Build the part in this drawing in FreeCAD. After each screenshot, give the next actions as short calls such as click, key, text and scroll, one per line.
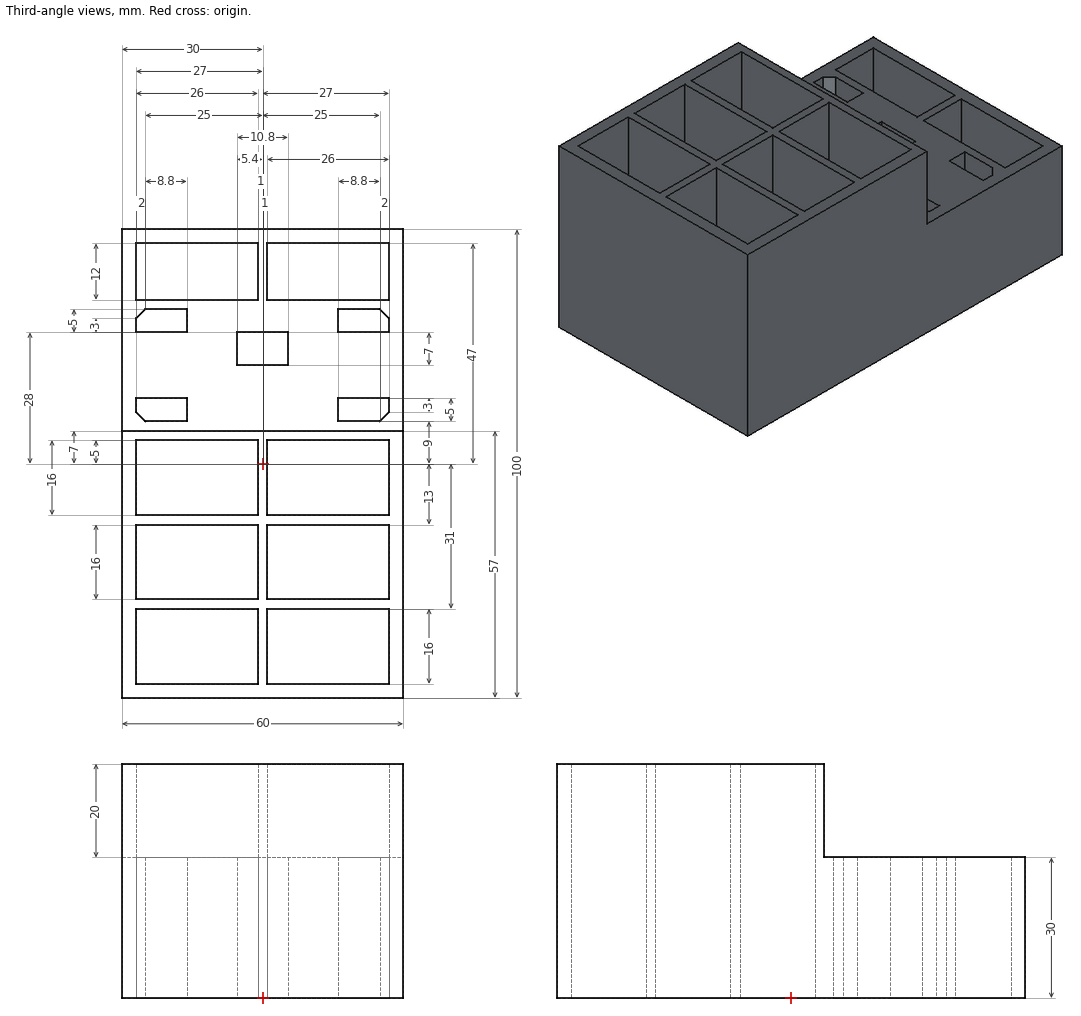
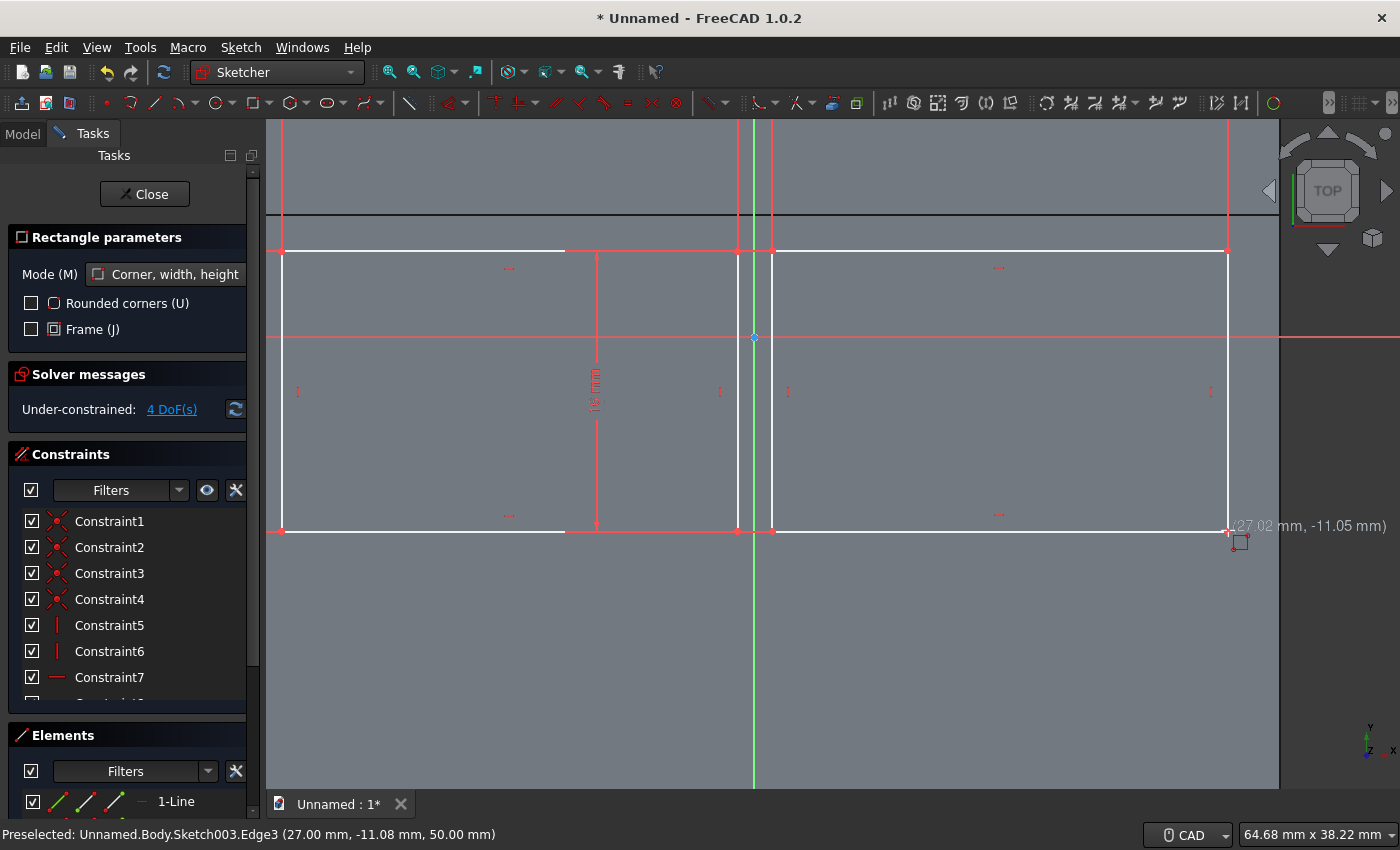
click(772, 565)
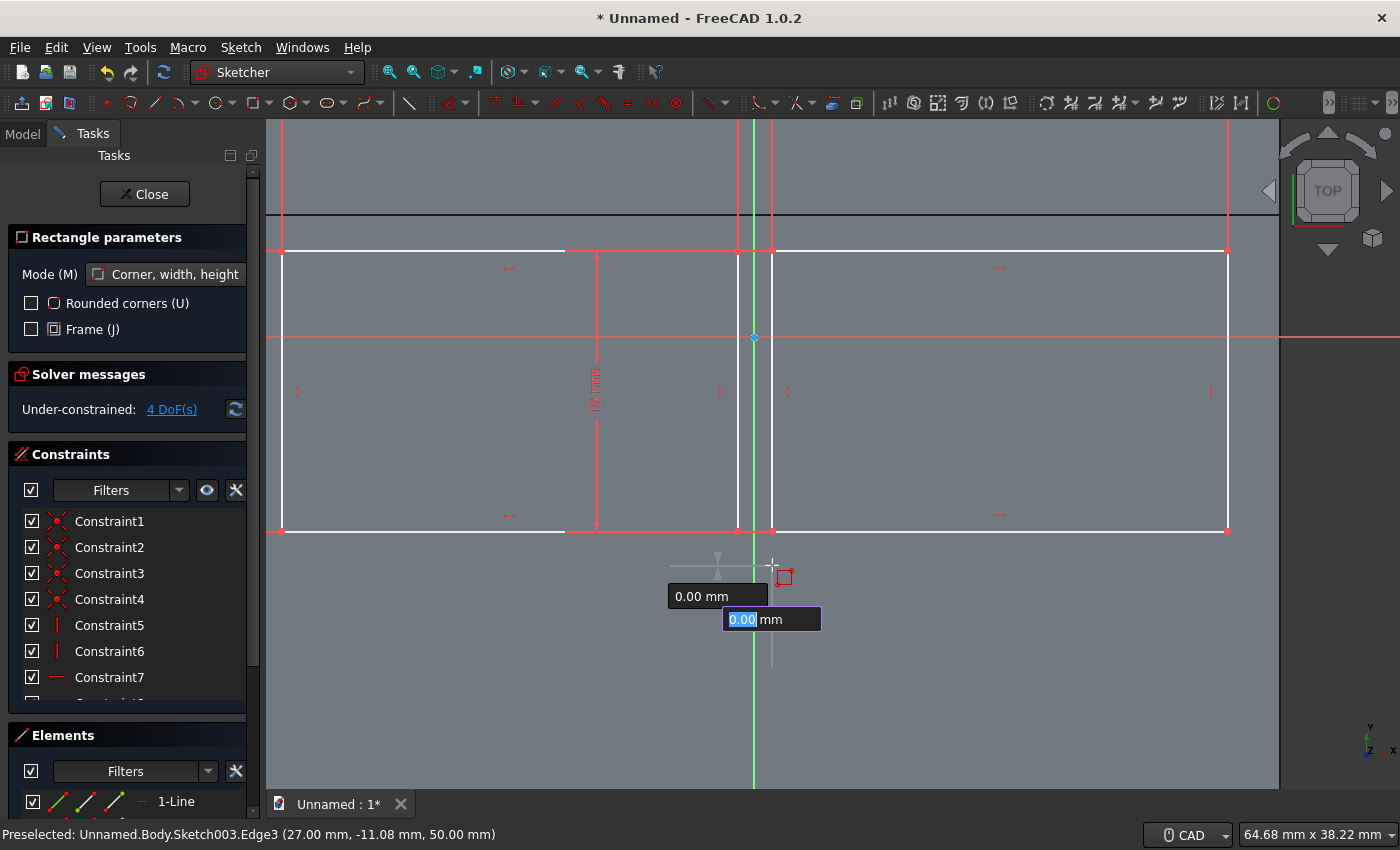
scroll(773, 249, down, 4)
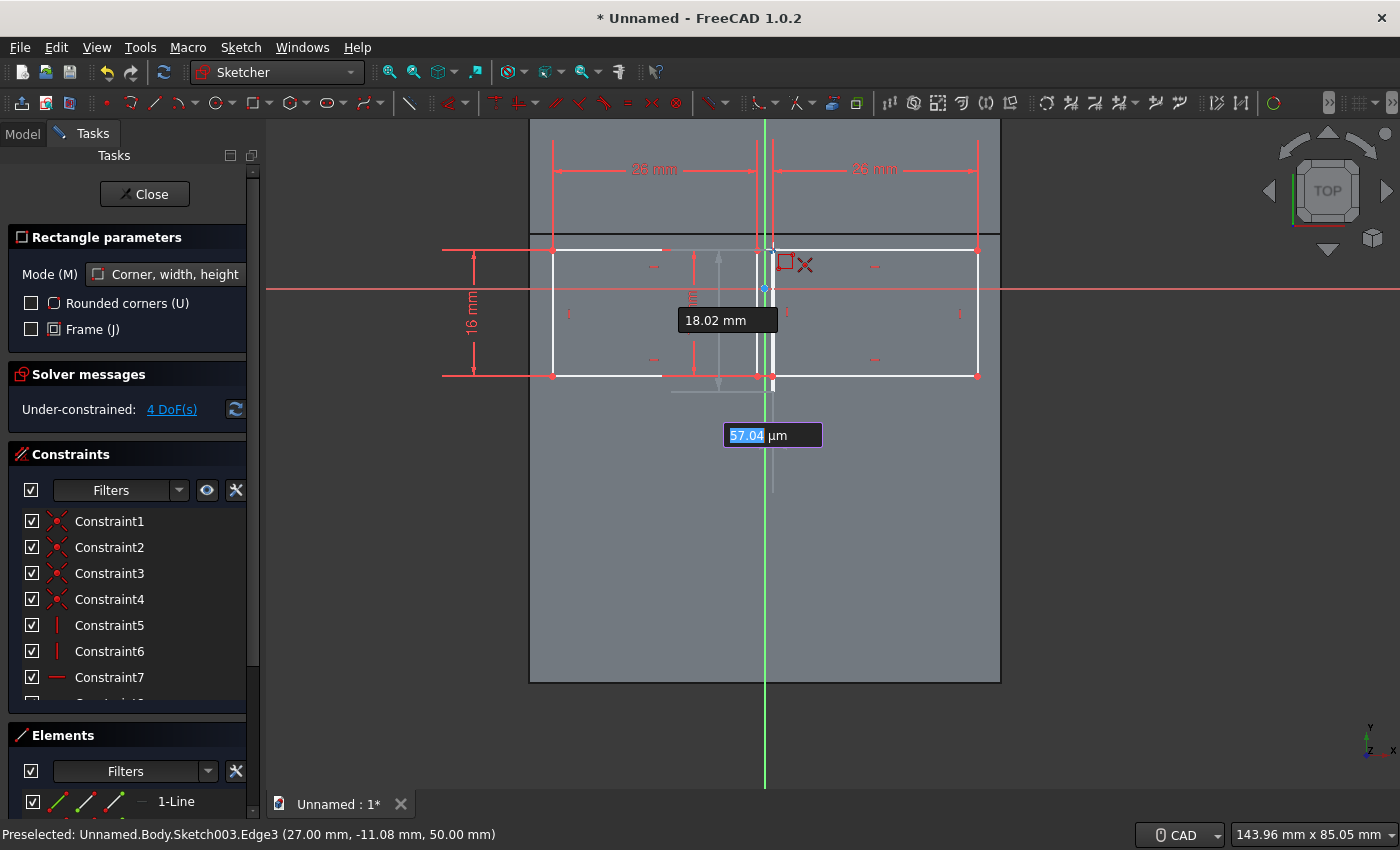
click(978, 517)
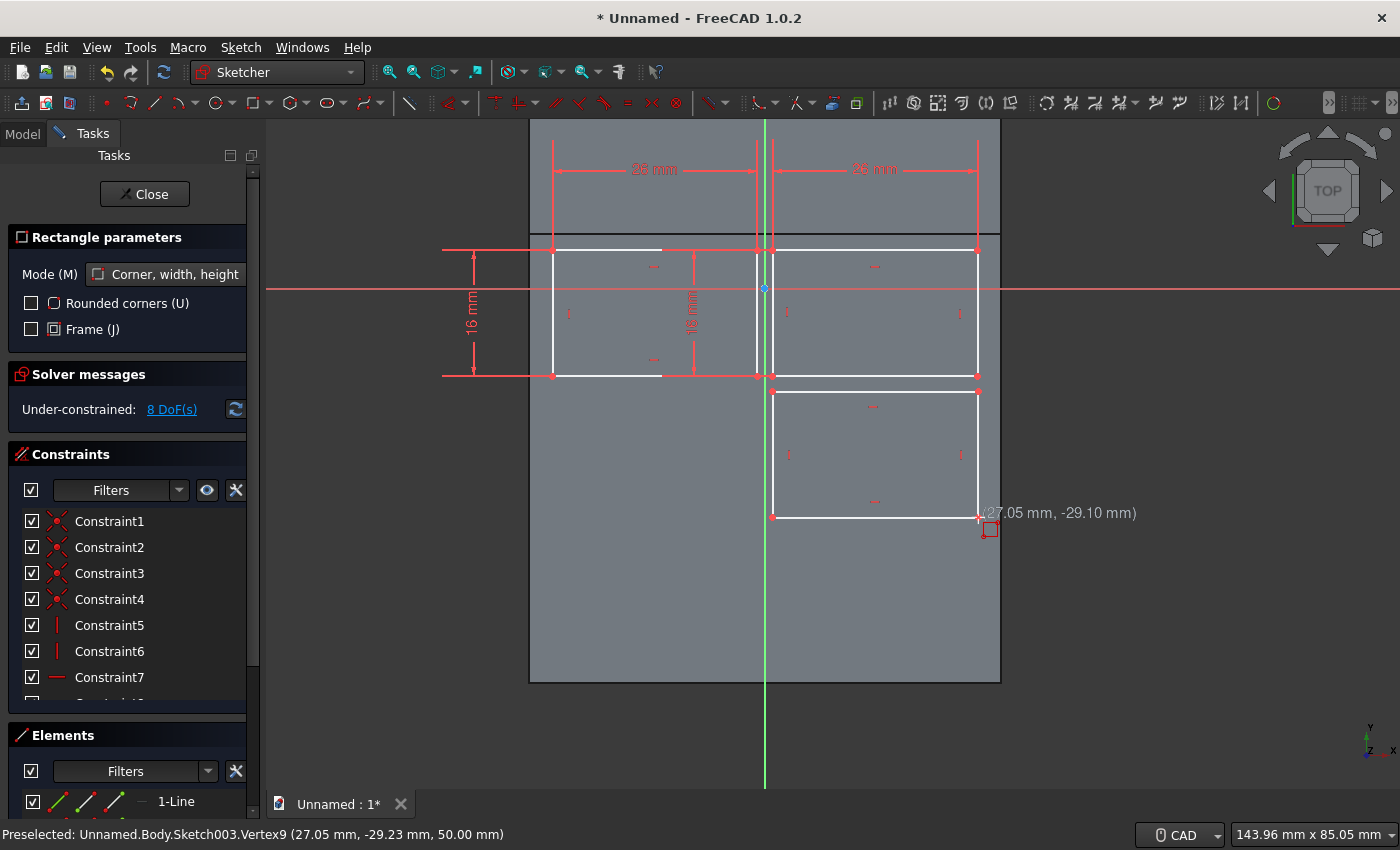
scroll(773, 533, up, 4)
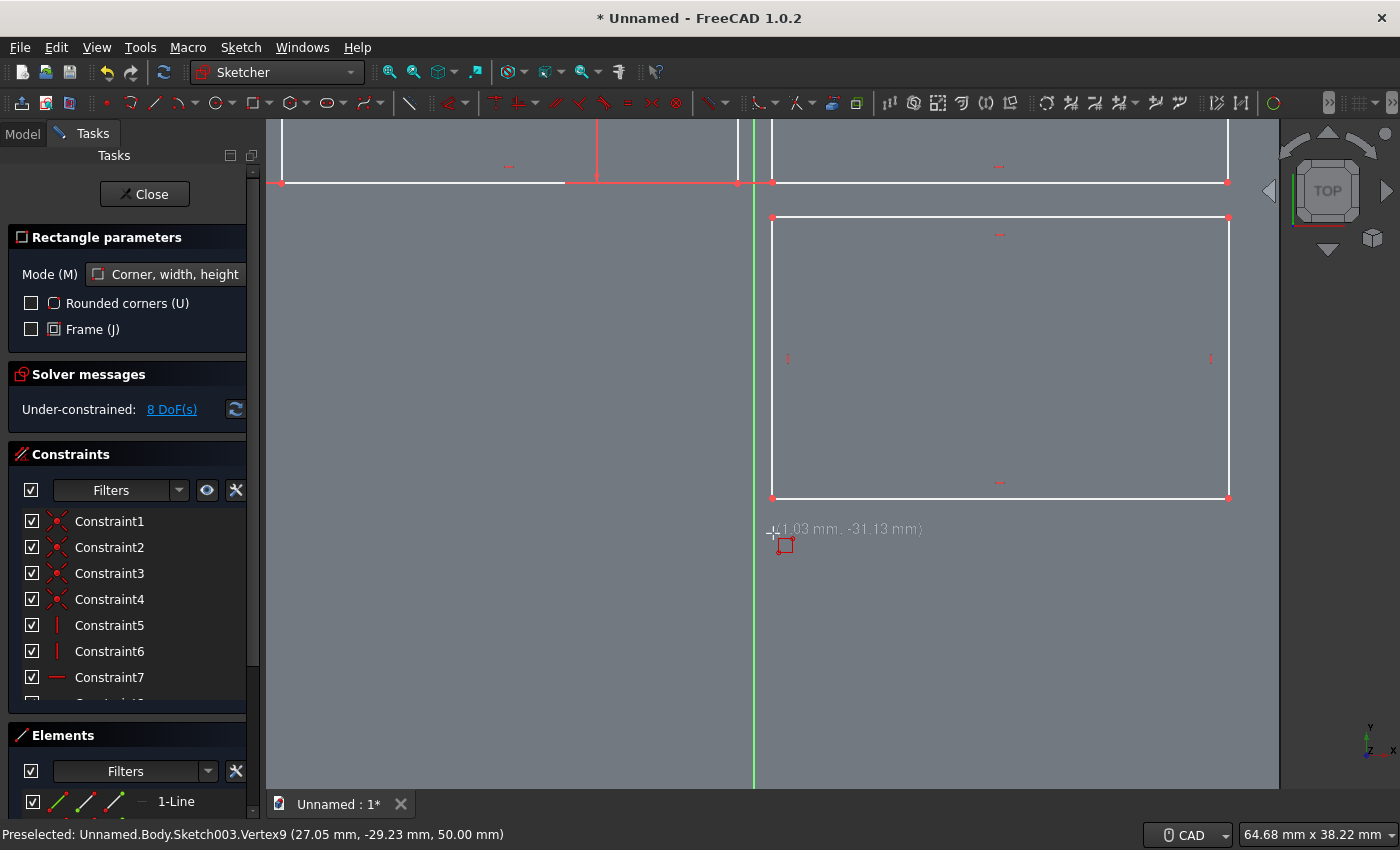
click(772, 532)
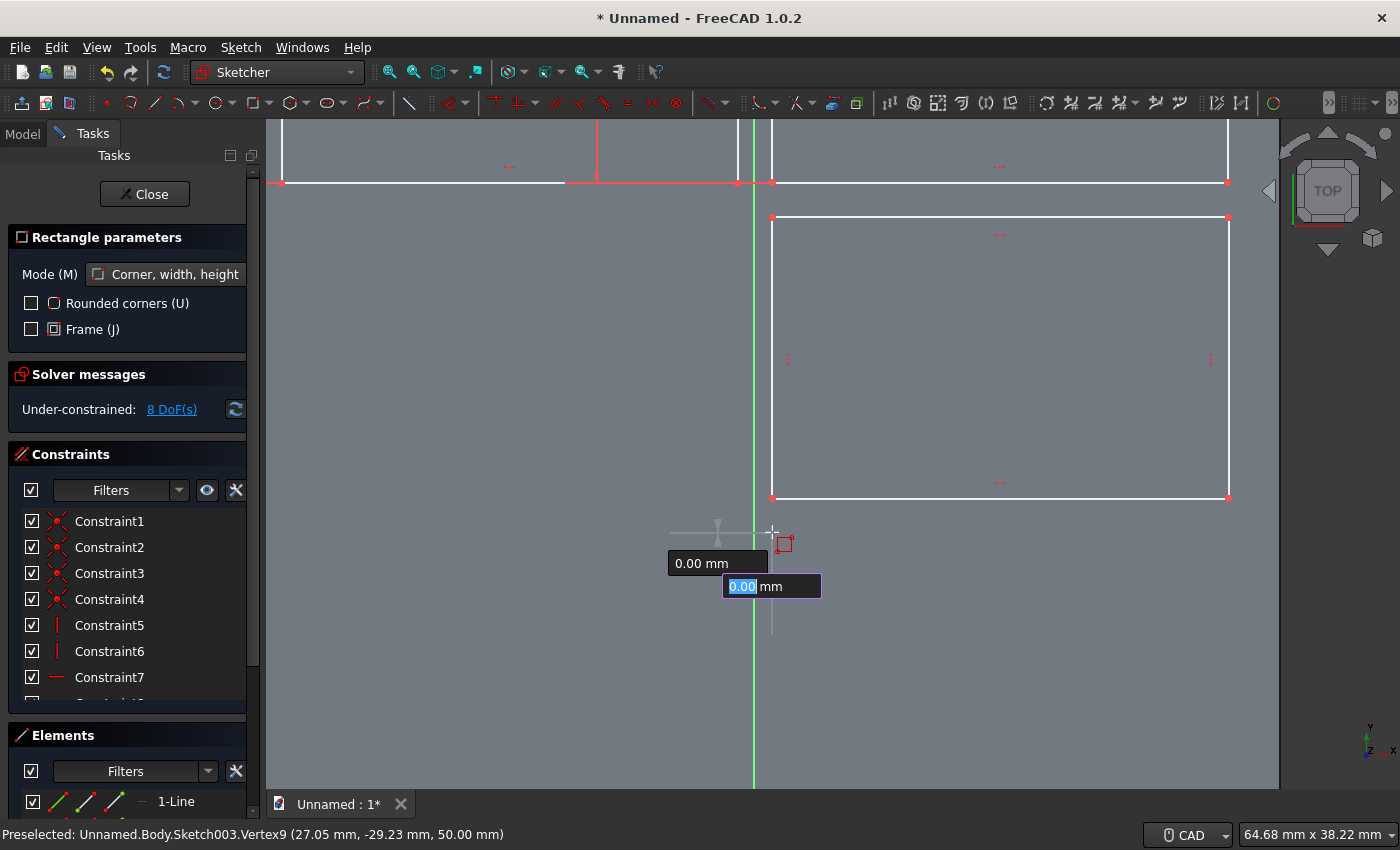
scroll(773, 533, down, 4)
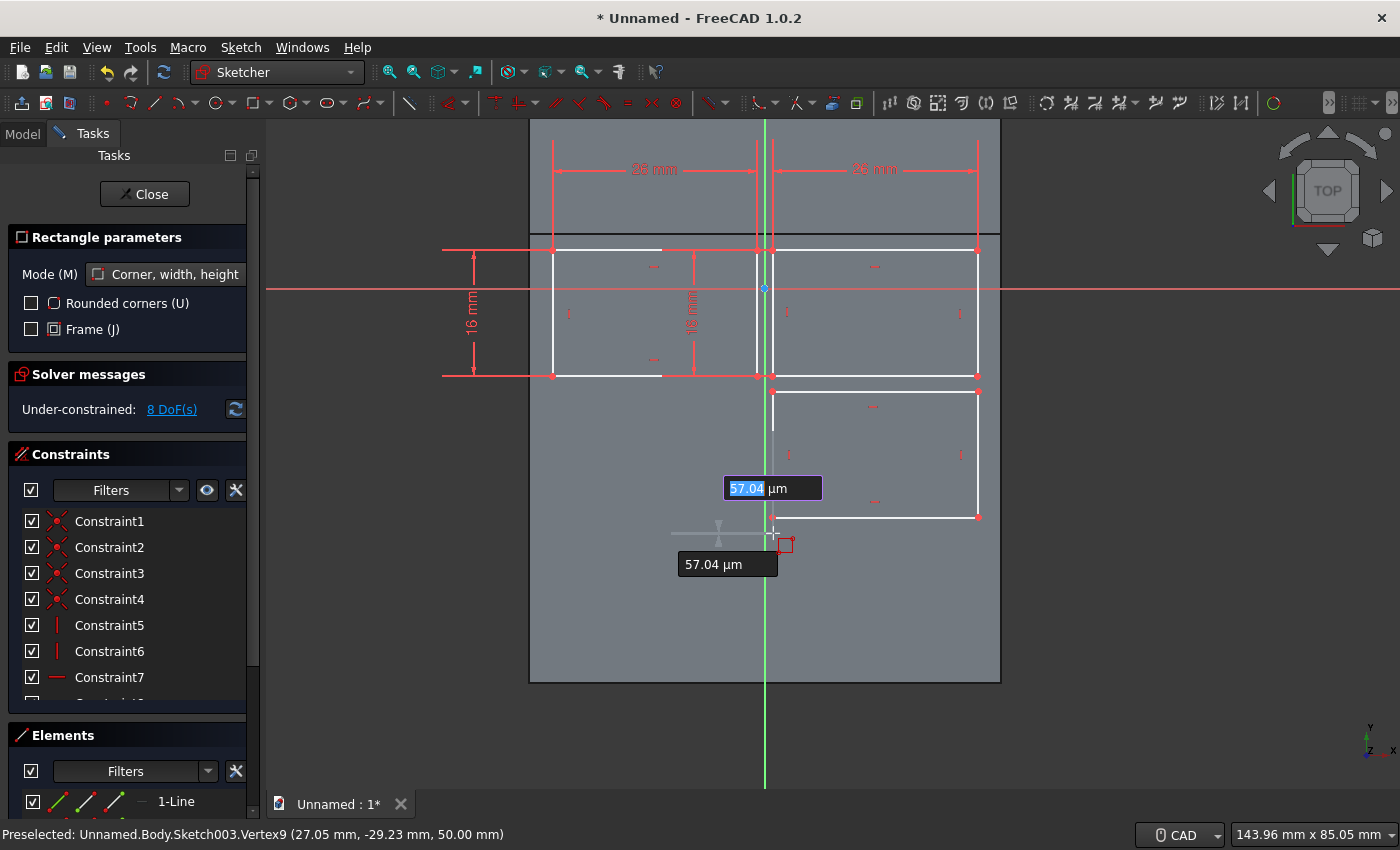
click(978, 659)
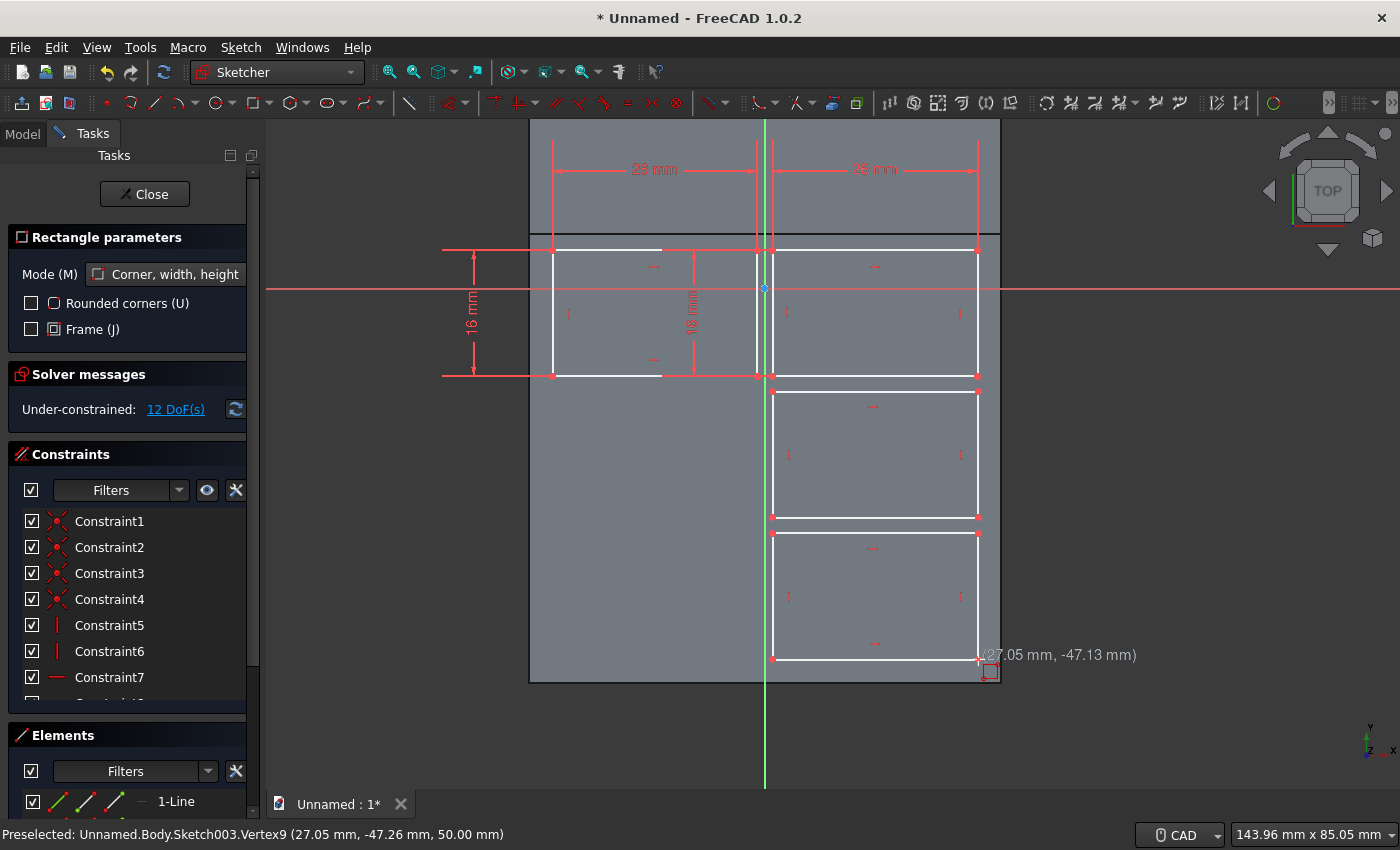
click(552, 391)